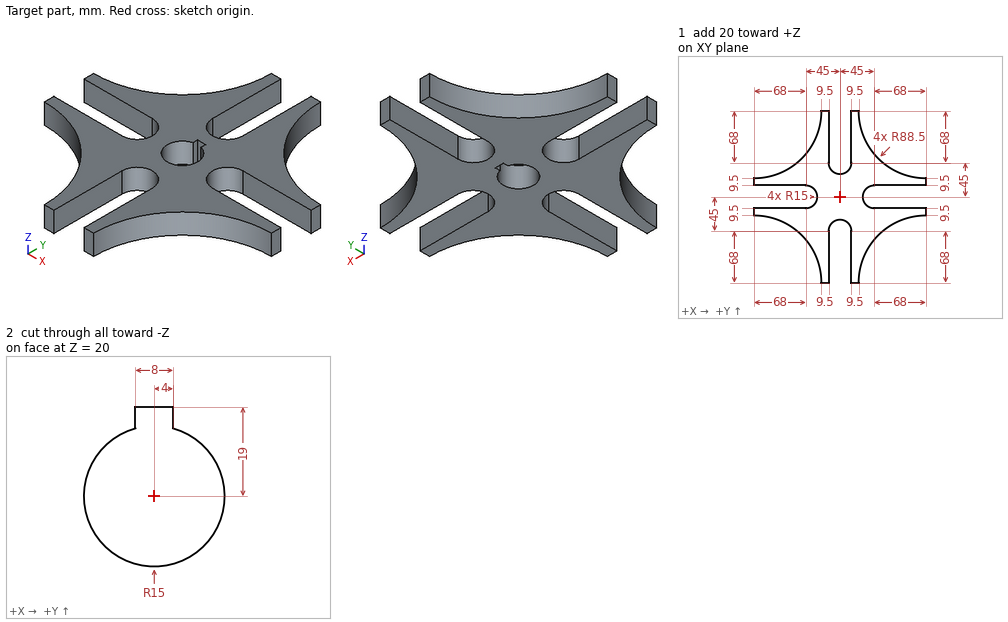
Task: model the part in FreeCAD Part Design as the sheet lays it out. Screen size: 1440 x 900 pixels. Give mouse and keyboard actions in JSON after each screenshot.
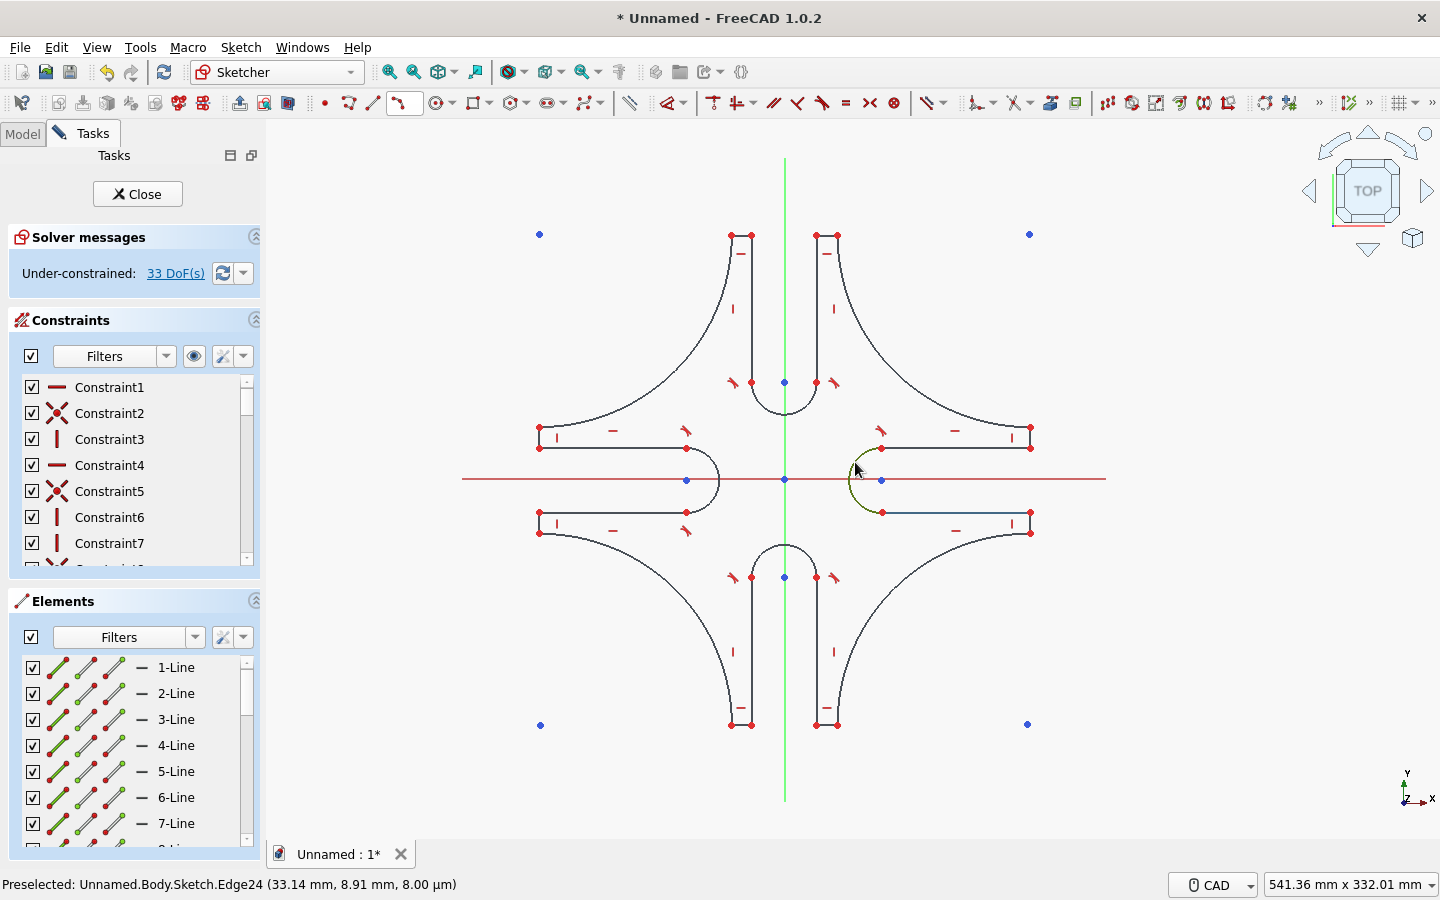
{"action": "left_click", "coordinate": [822, 104]}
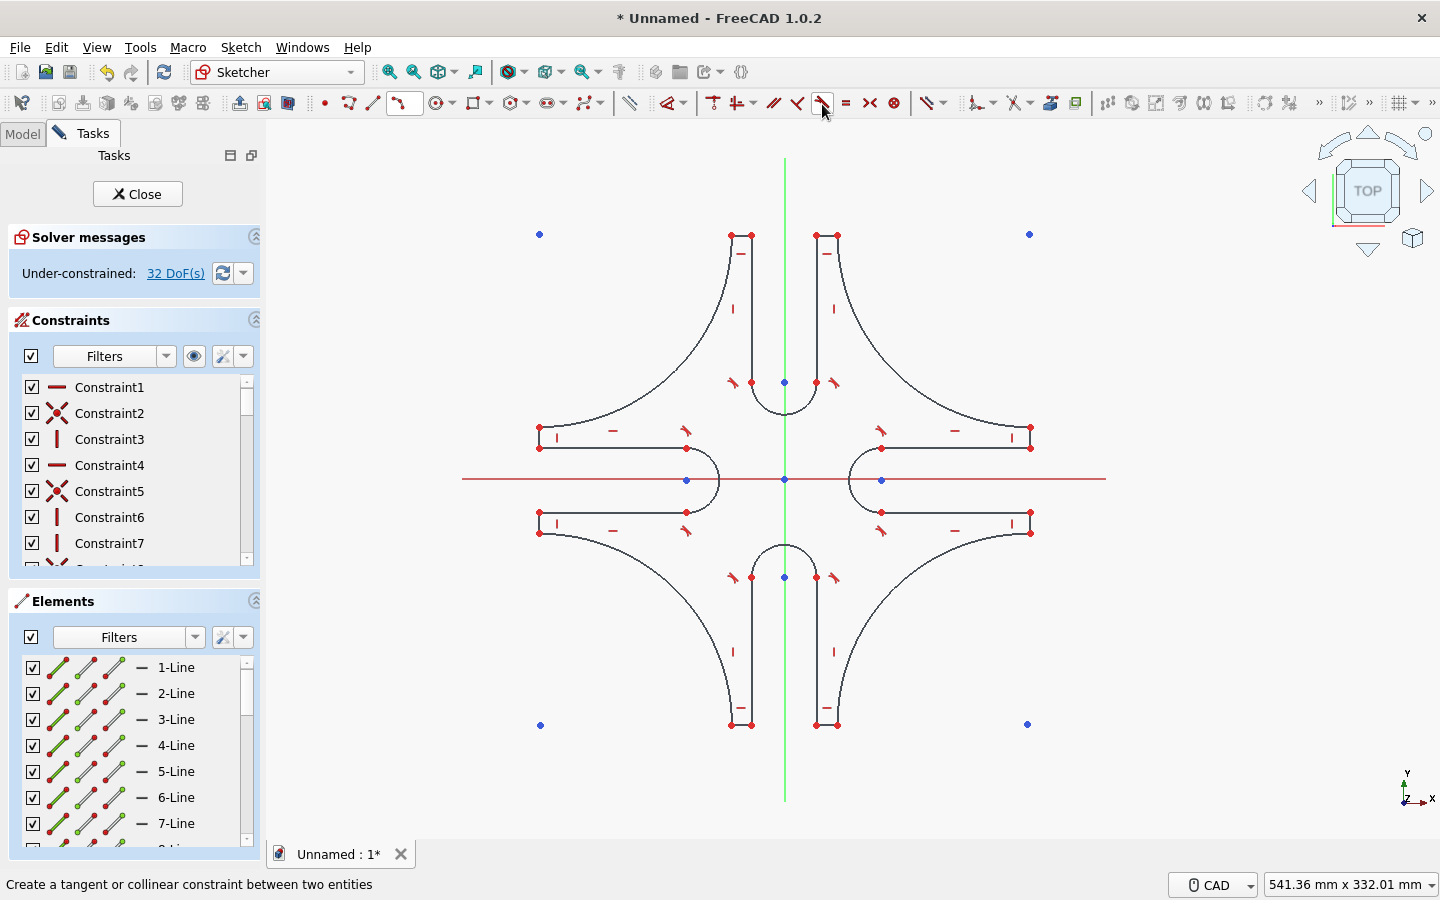
{"action": "left_click", "coordinate": [859, 323]}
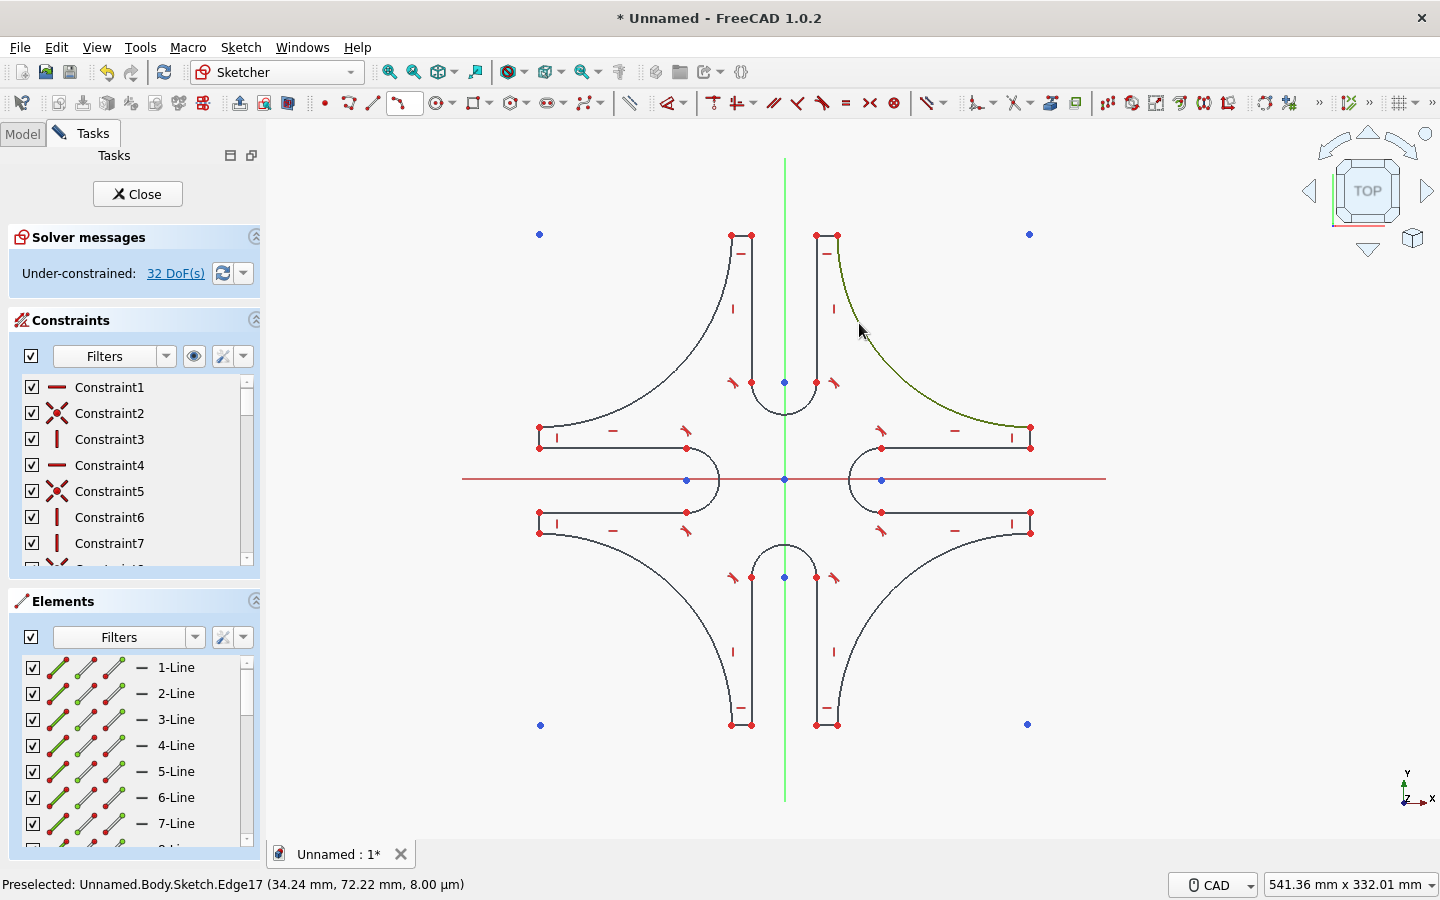
{"action": "left_click", "coordinate": [626, 406]}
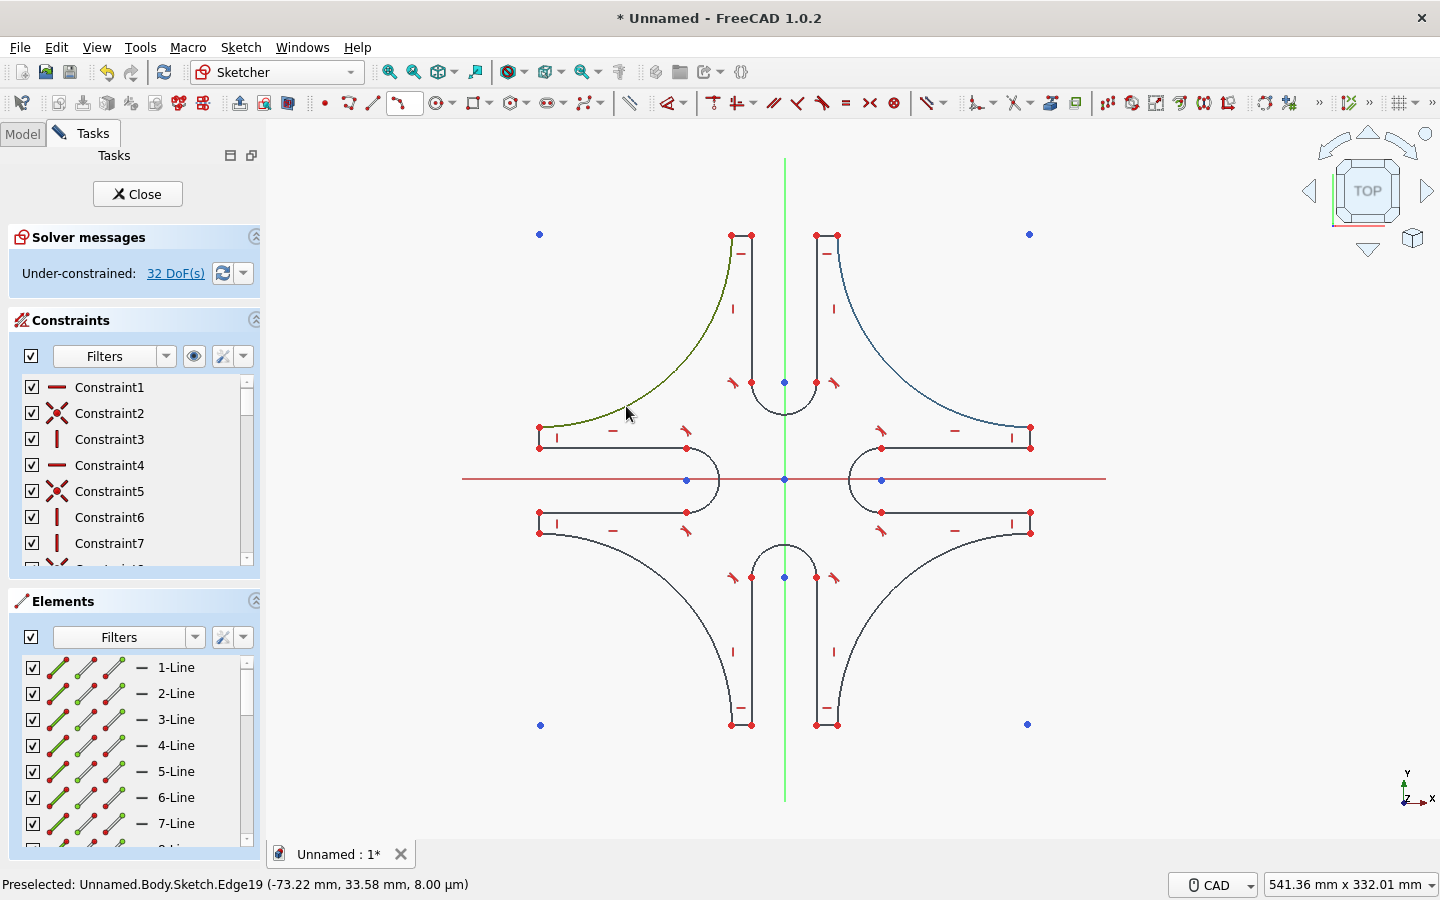
{"action": "left_click", "coordinate": [711, 638]}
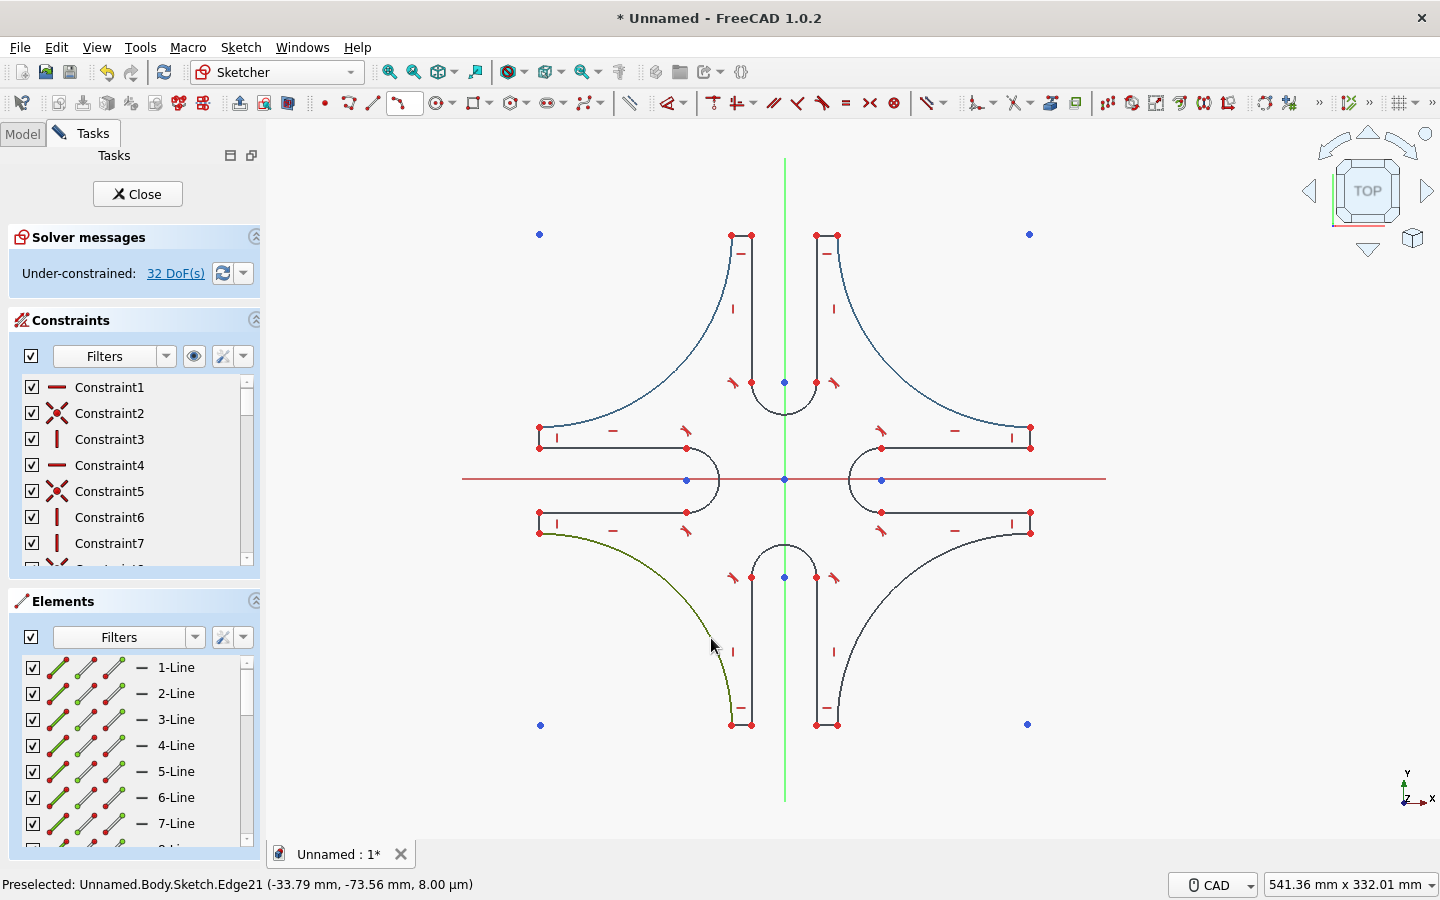
{"action": "left_click", "coordinate": [943, 554]}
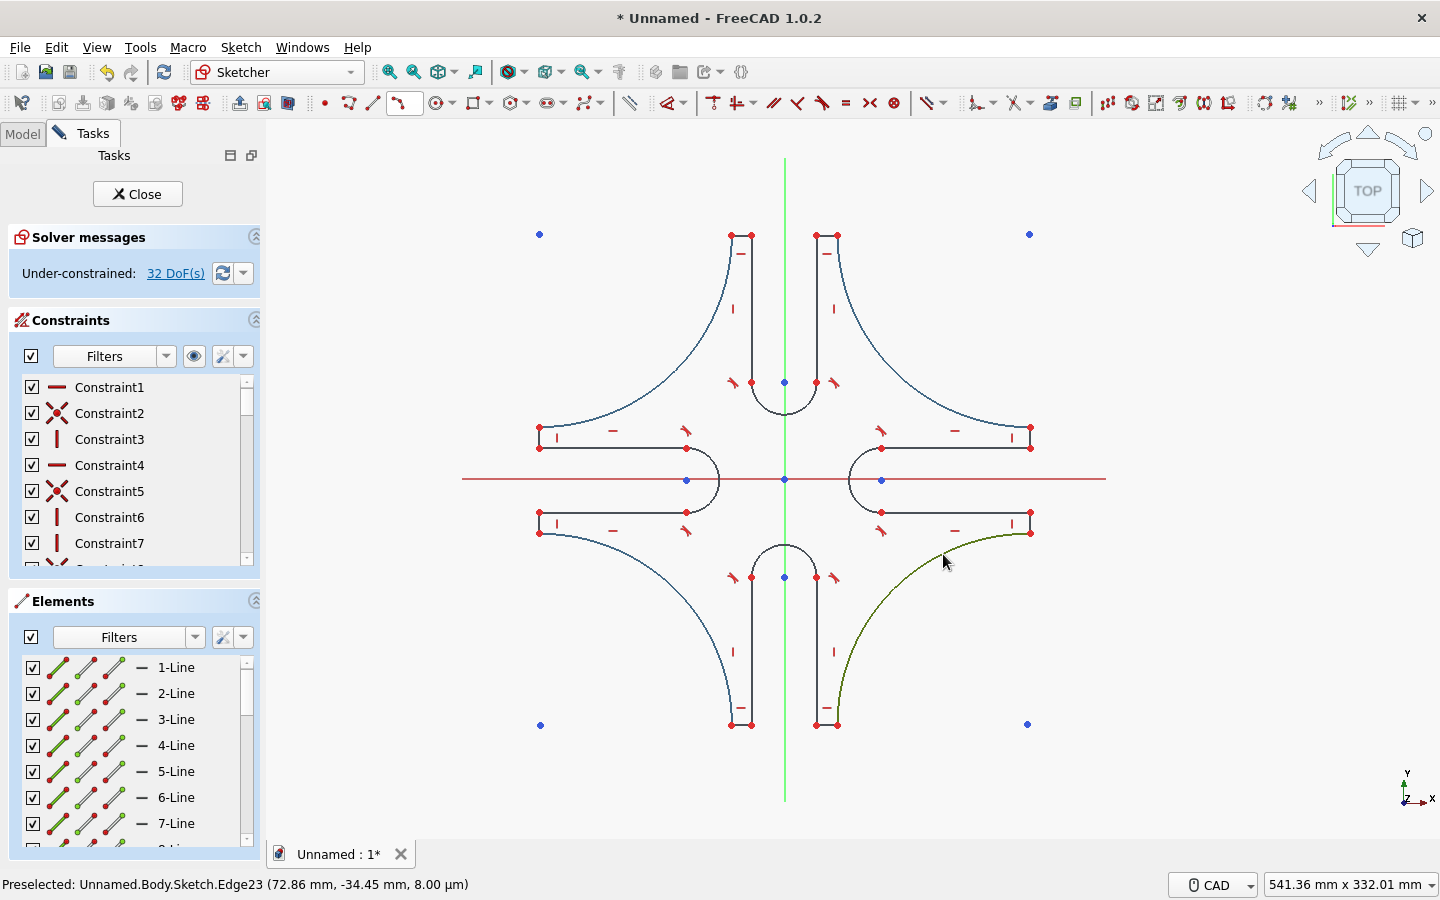
{"action": "left_click", "coordinate": [846, 104]}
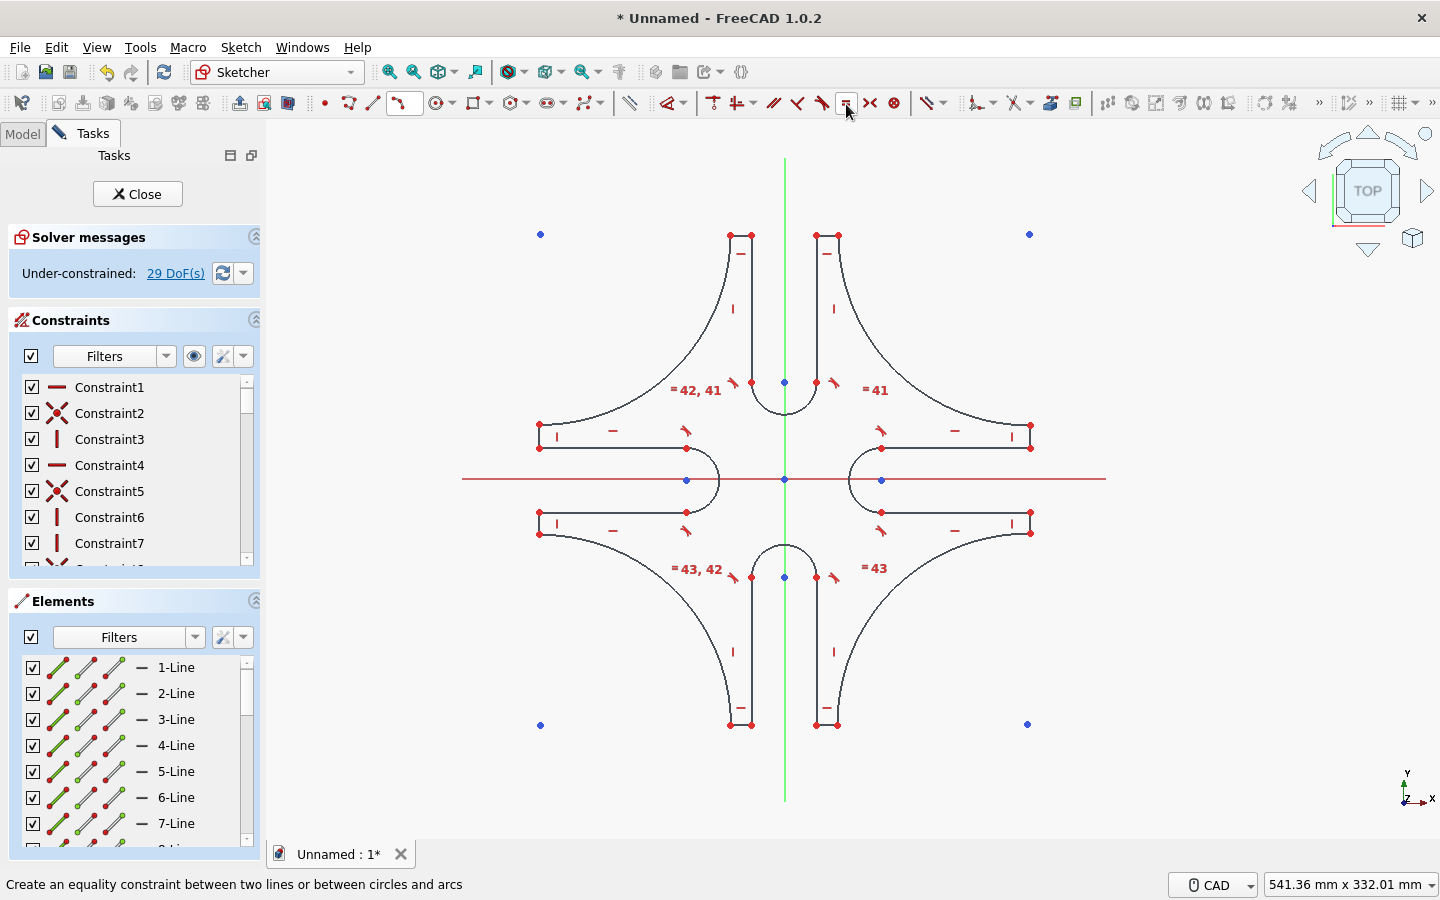
{"action": "left_click", "coordinate": [765, 408]}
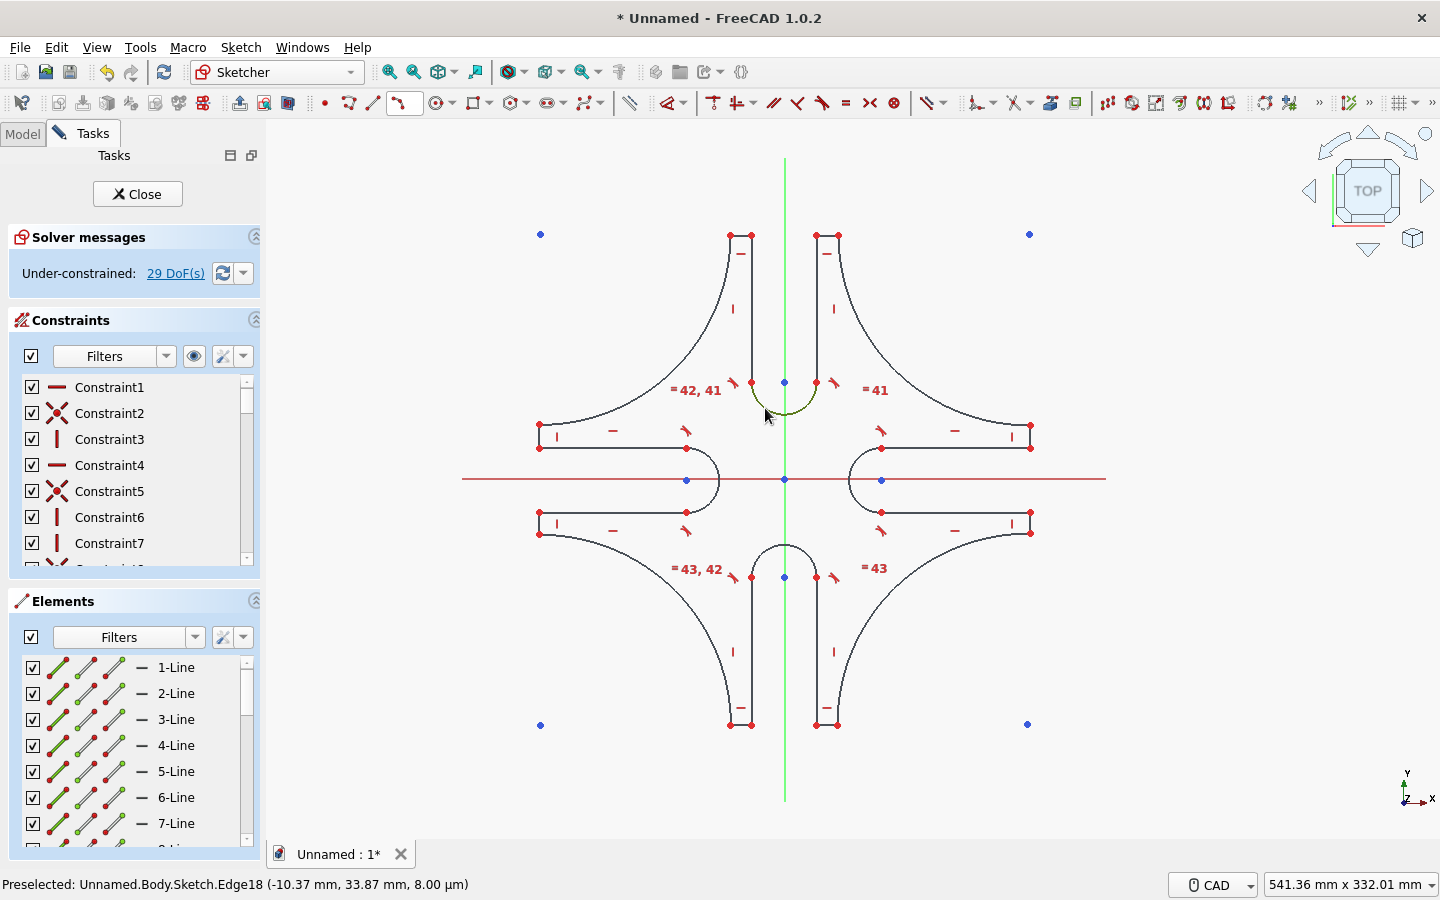
{"action": "left_click", "coordinate": [713, 500]}